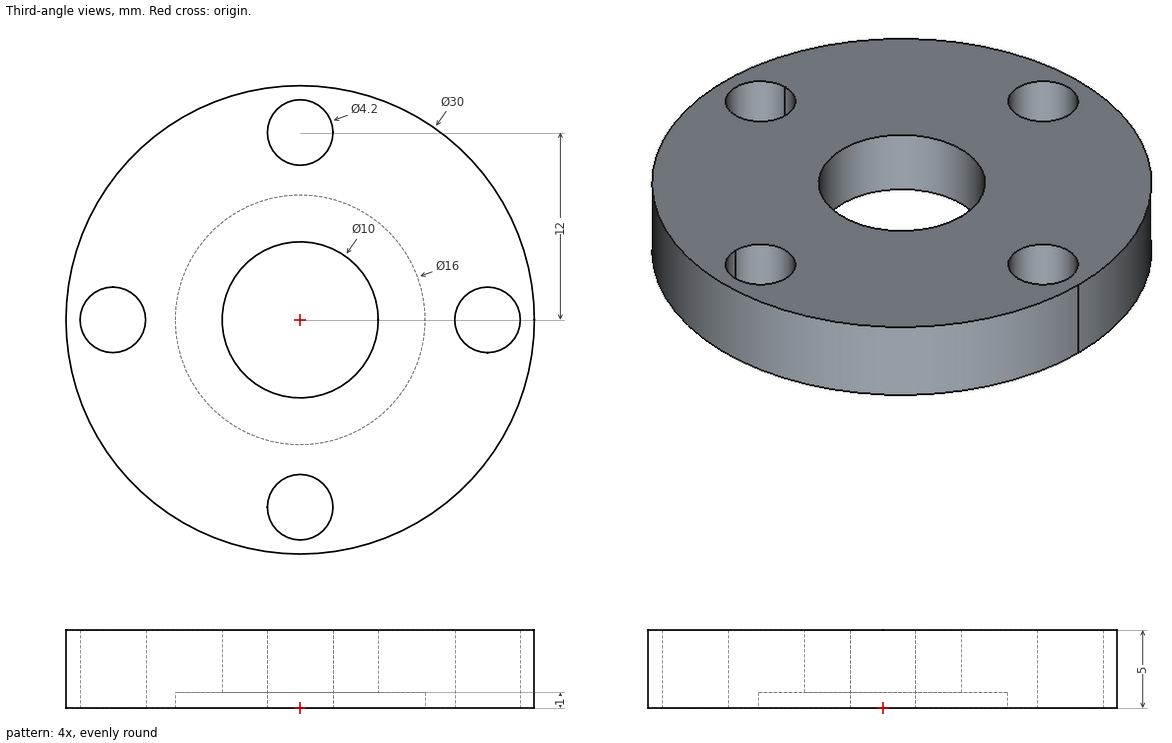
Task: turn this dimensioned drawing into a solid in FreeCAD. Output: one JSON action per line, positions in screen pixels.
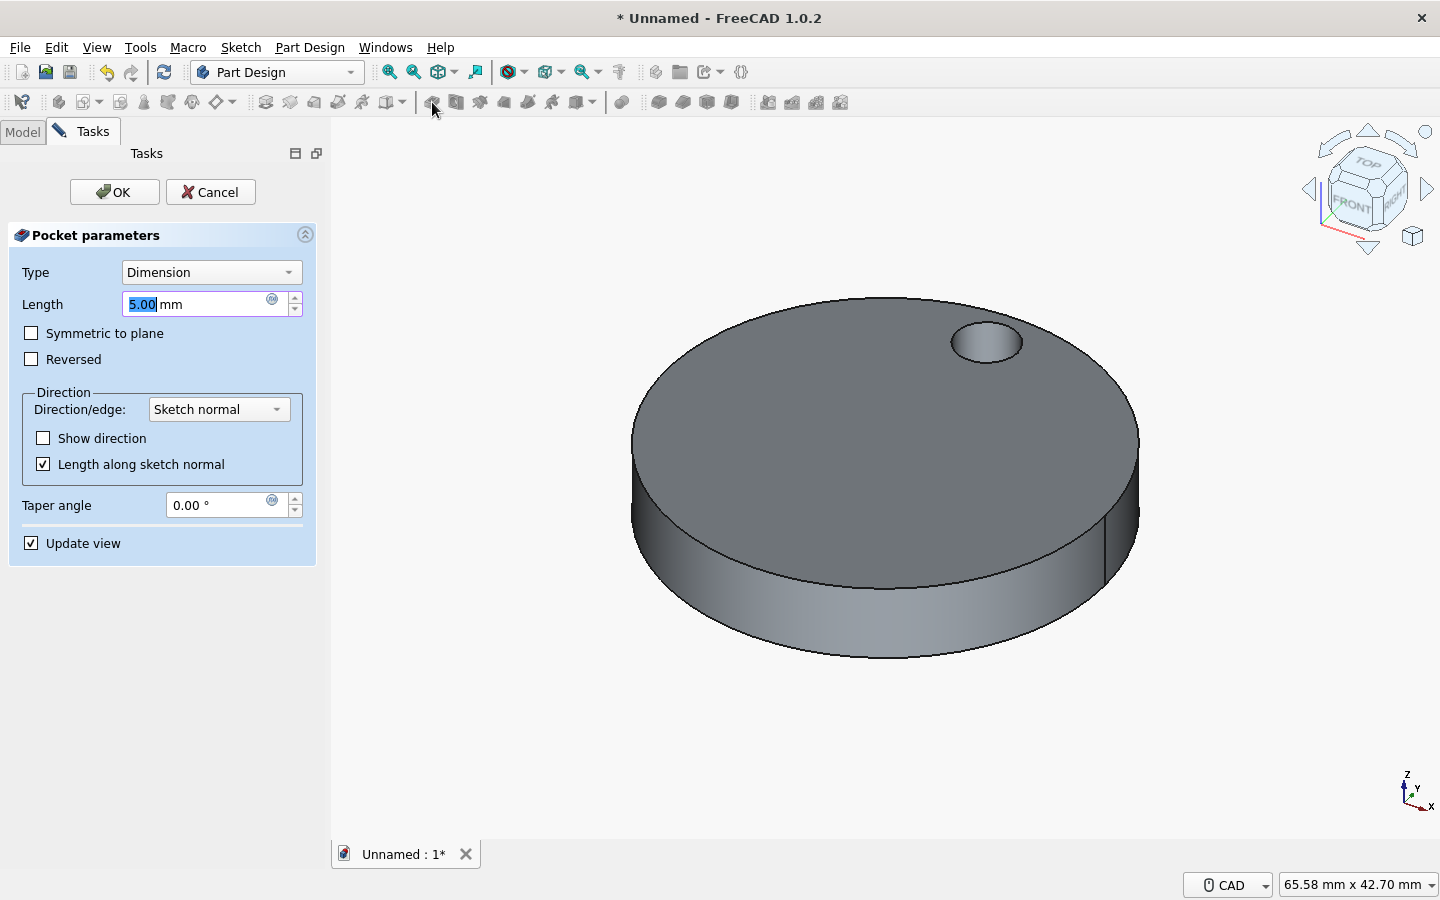
{"action": "left_click", "coordinate": [212, 272]}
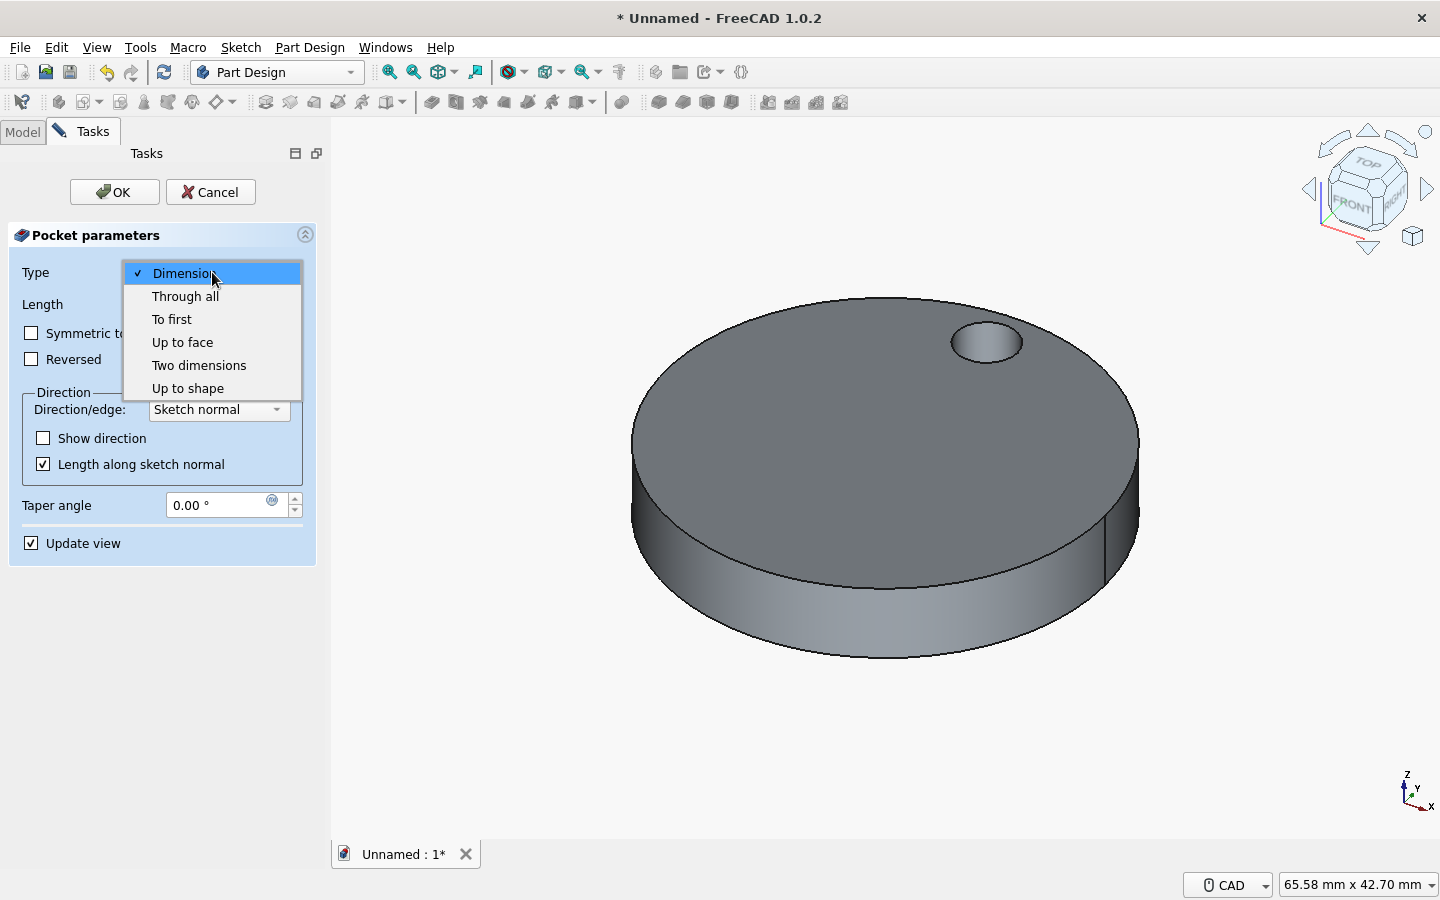
{"action": "left_click", "coordinate": [212, 296]}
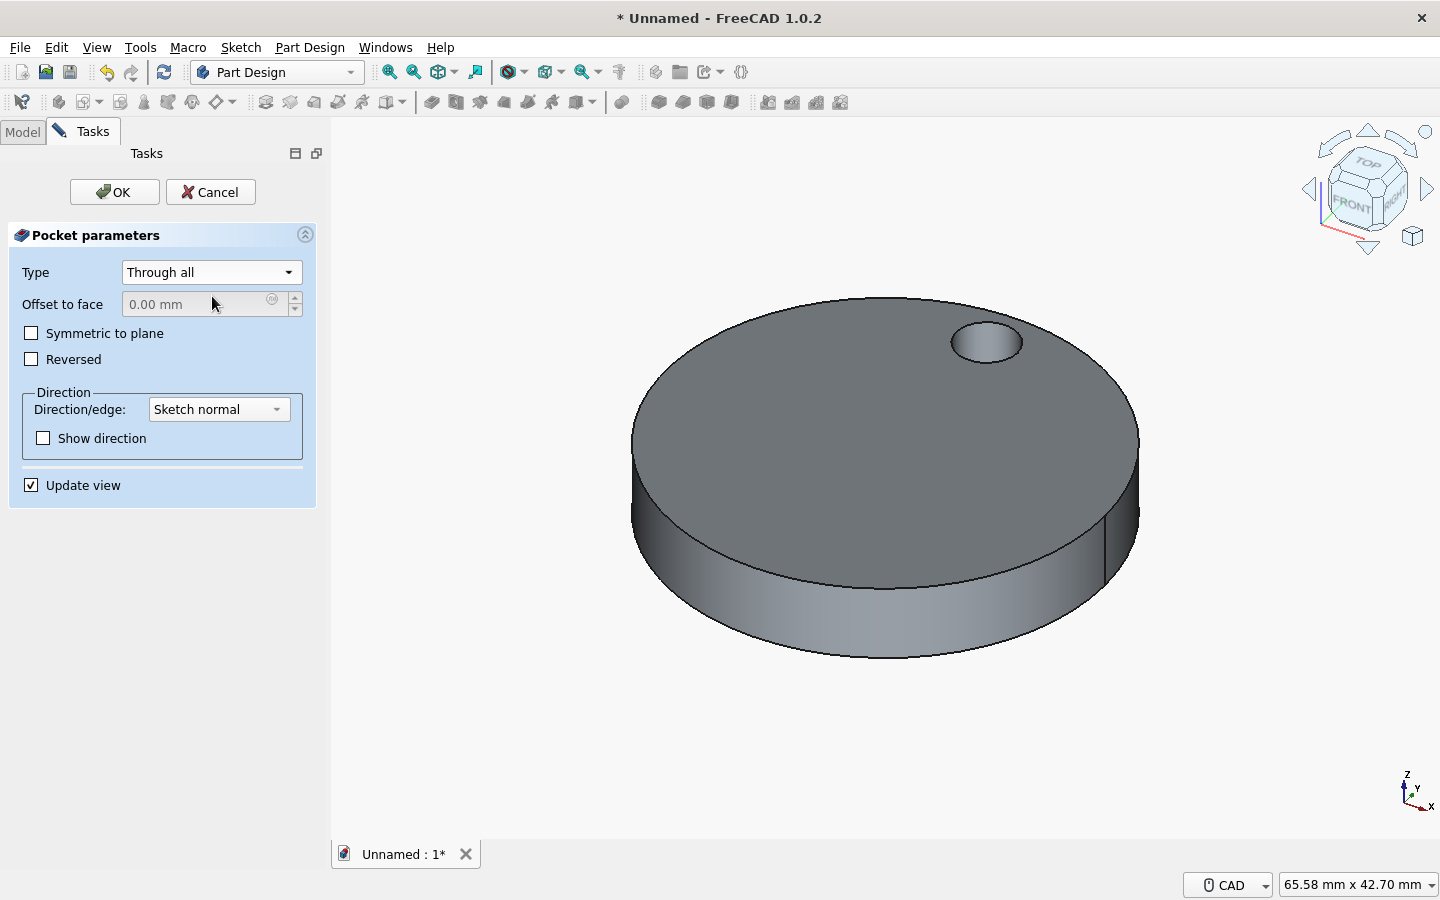
{"action": "left_click", "coordinate": [115, 192]}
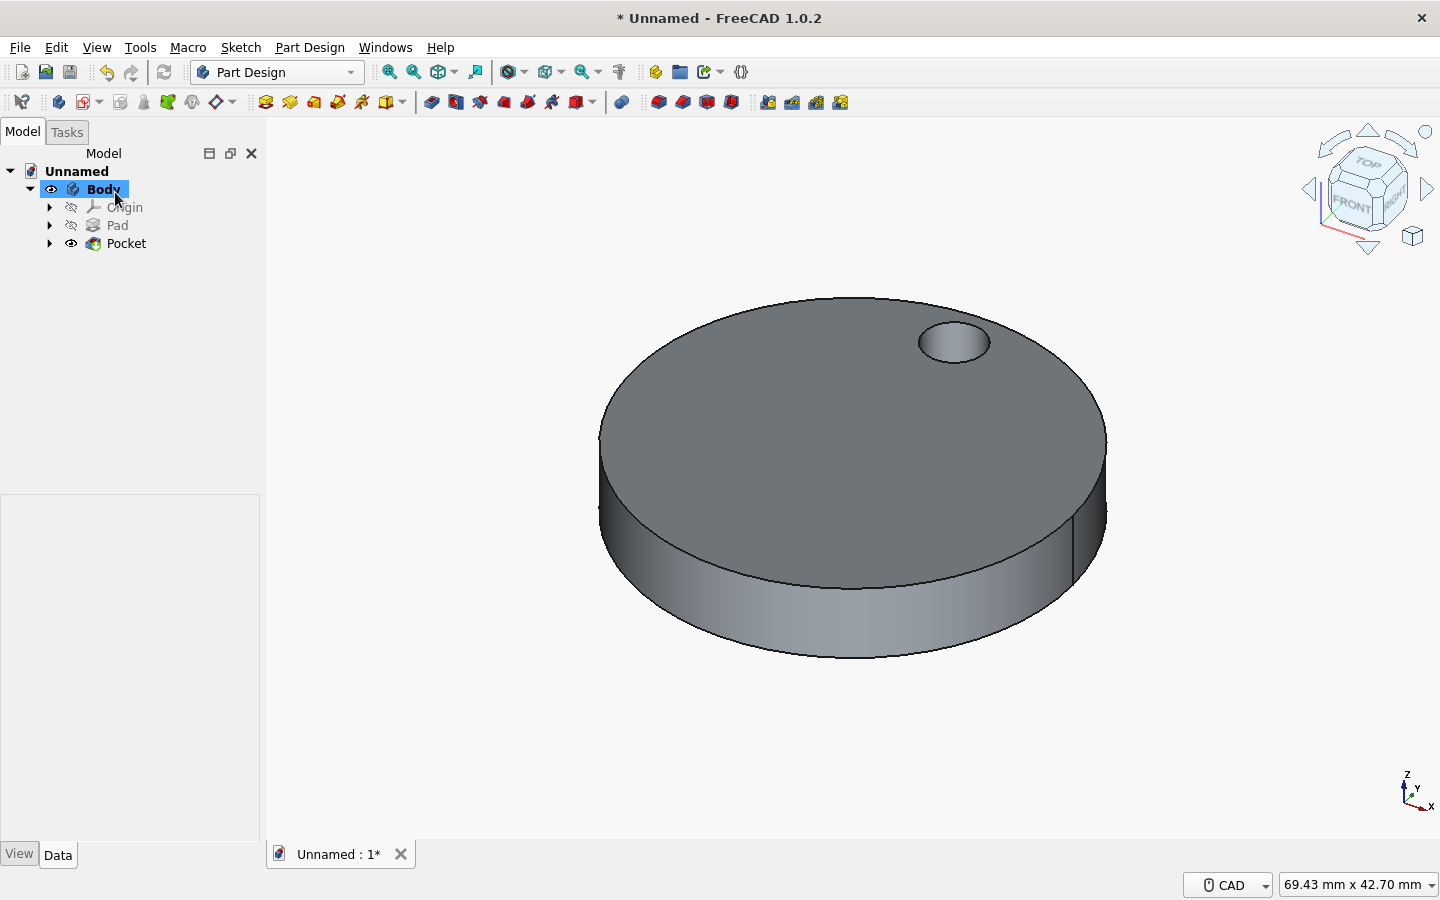
{"action": "left_click", "coordinate": [116, 243]}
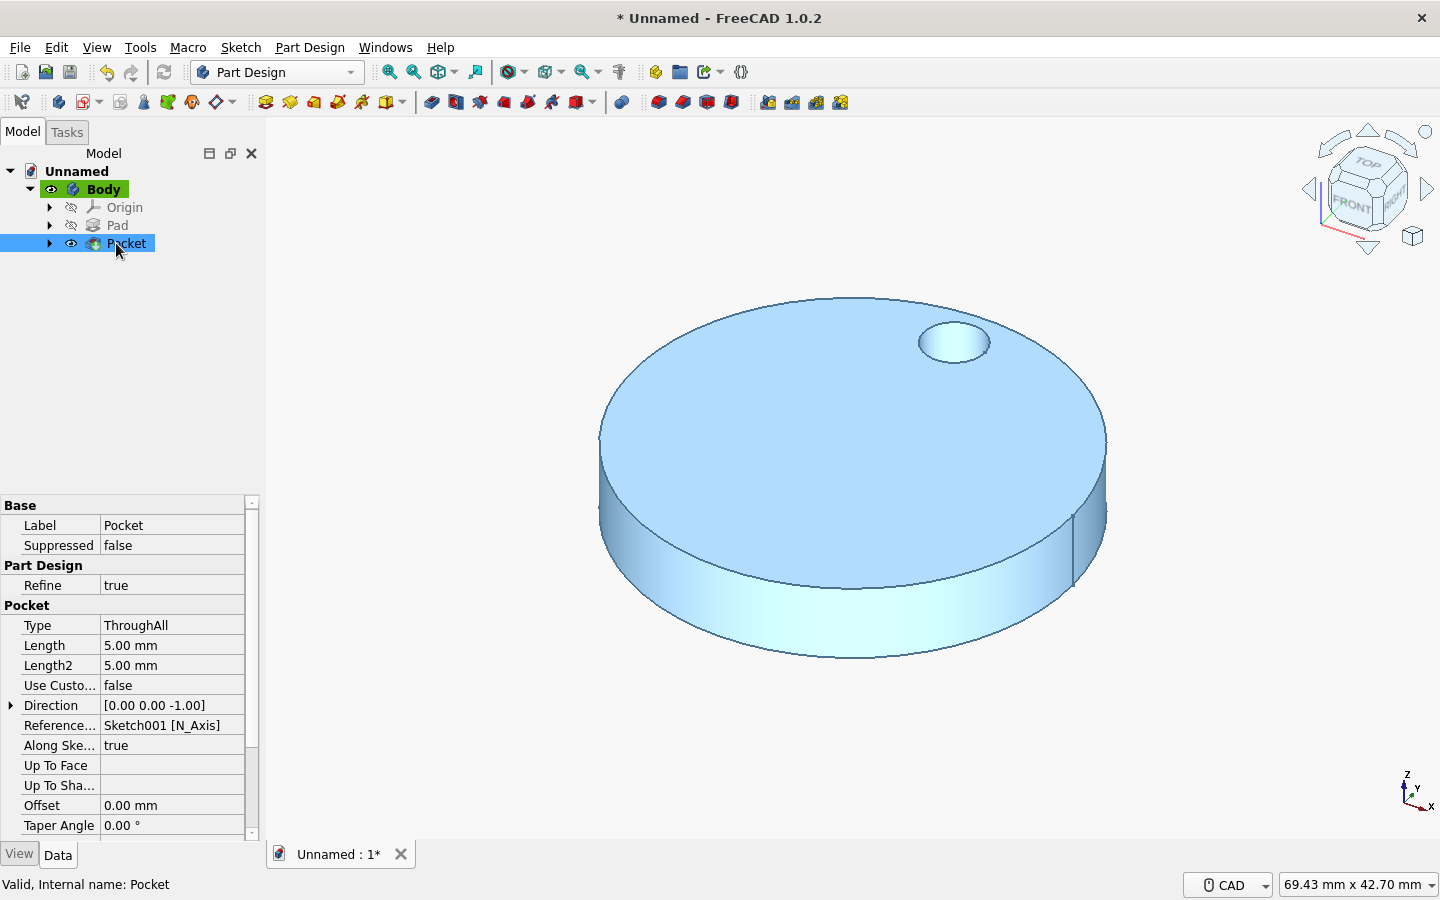
{"action": "left_click", "coordinate": [816, 102]}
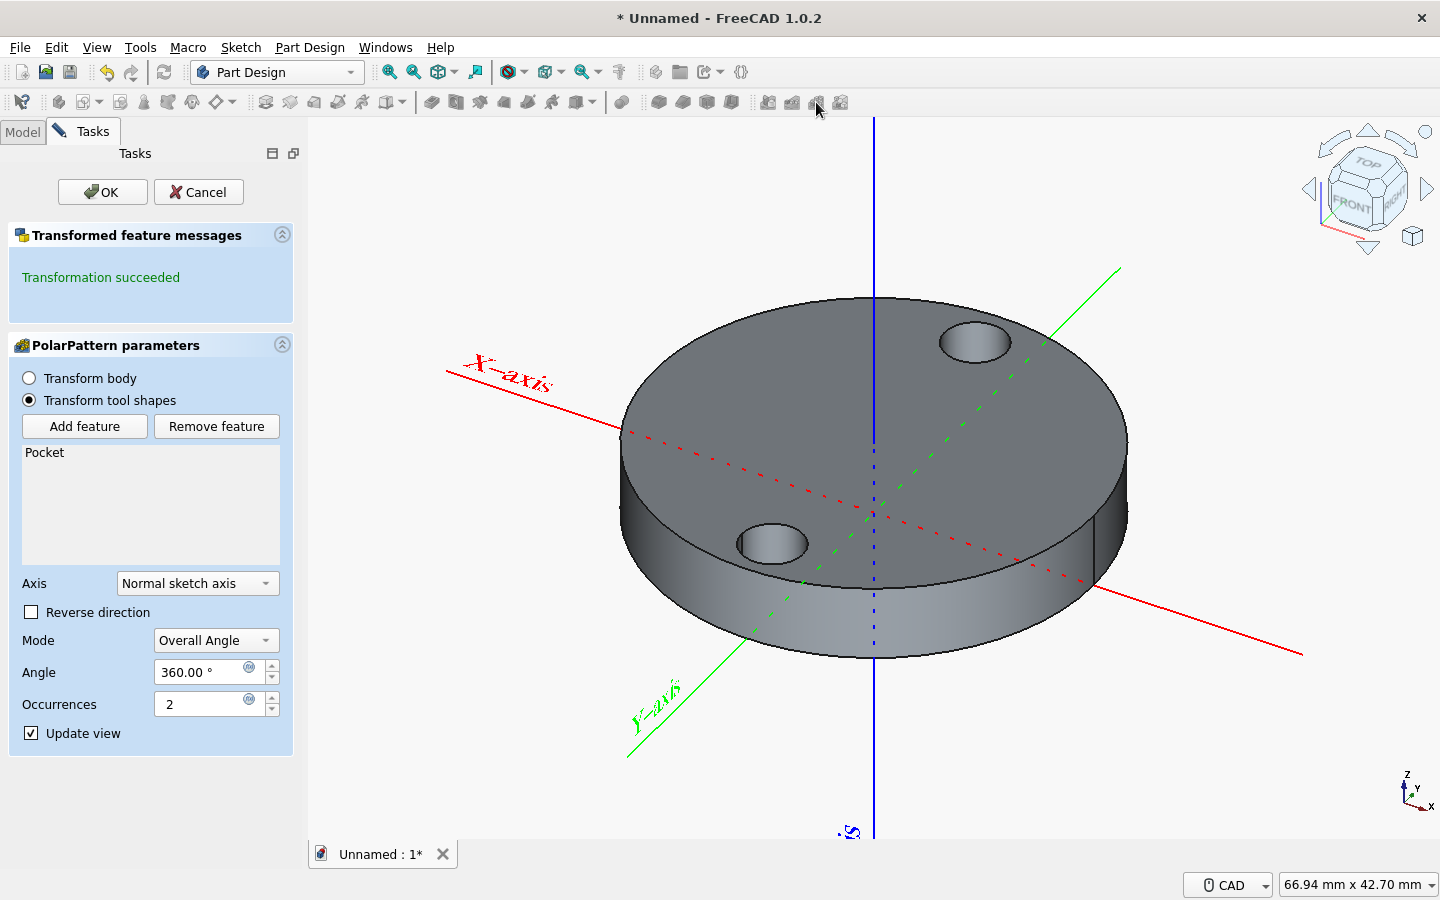
{"action": "left_click", "coordinate": [198, 584]}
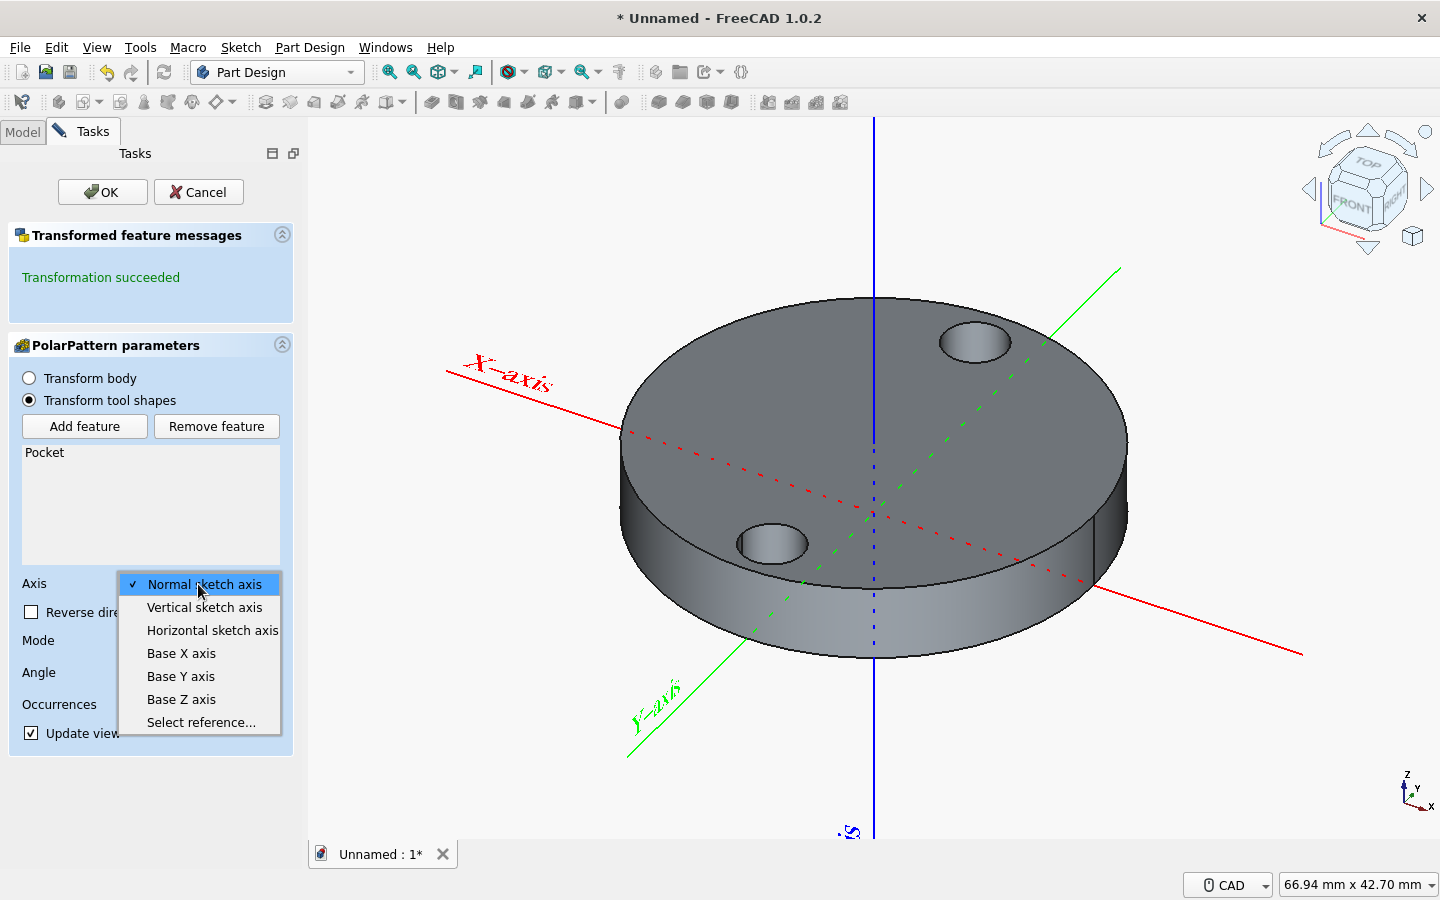
{"action": "left_click", "coordinate": [198, 700]}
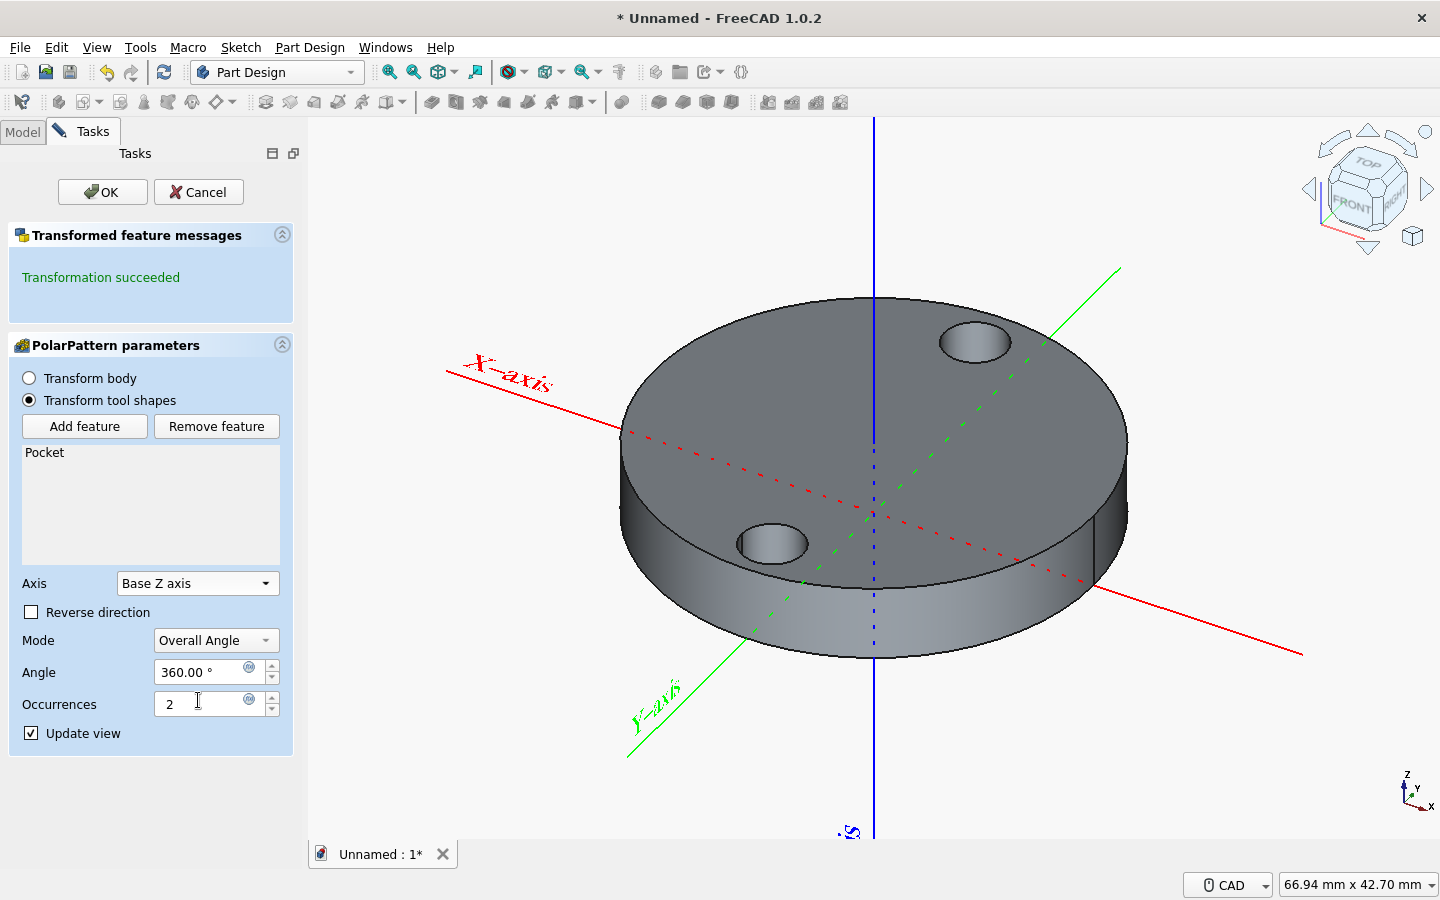
{"action": "triple_click", "coordinate": [209, 704]}